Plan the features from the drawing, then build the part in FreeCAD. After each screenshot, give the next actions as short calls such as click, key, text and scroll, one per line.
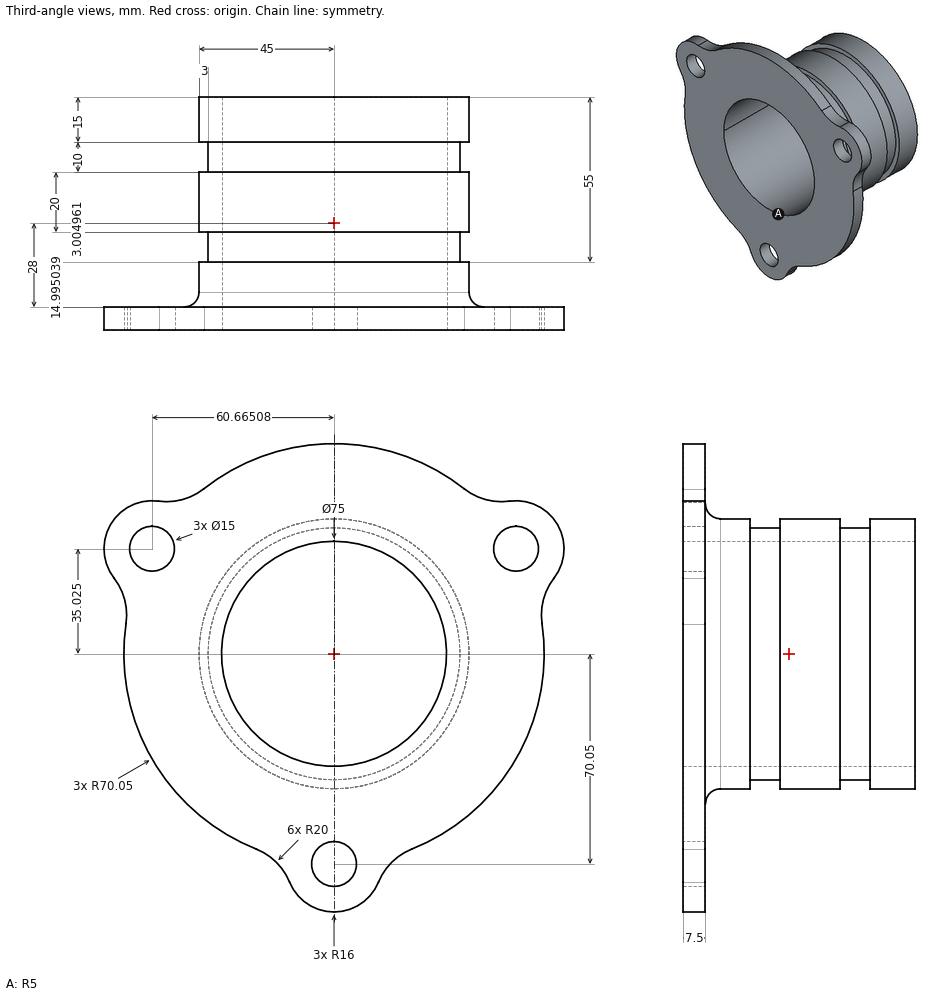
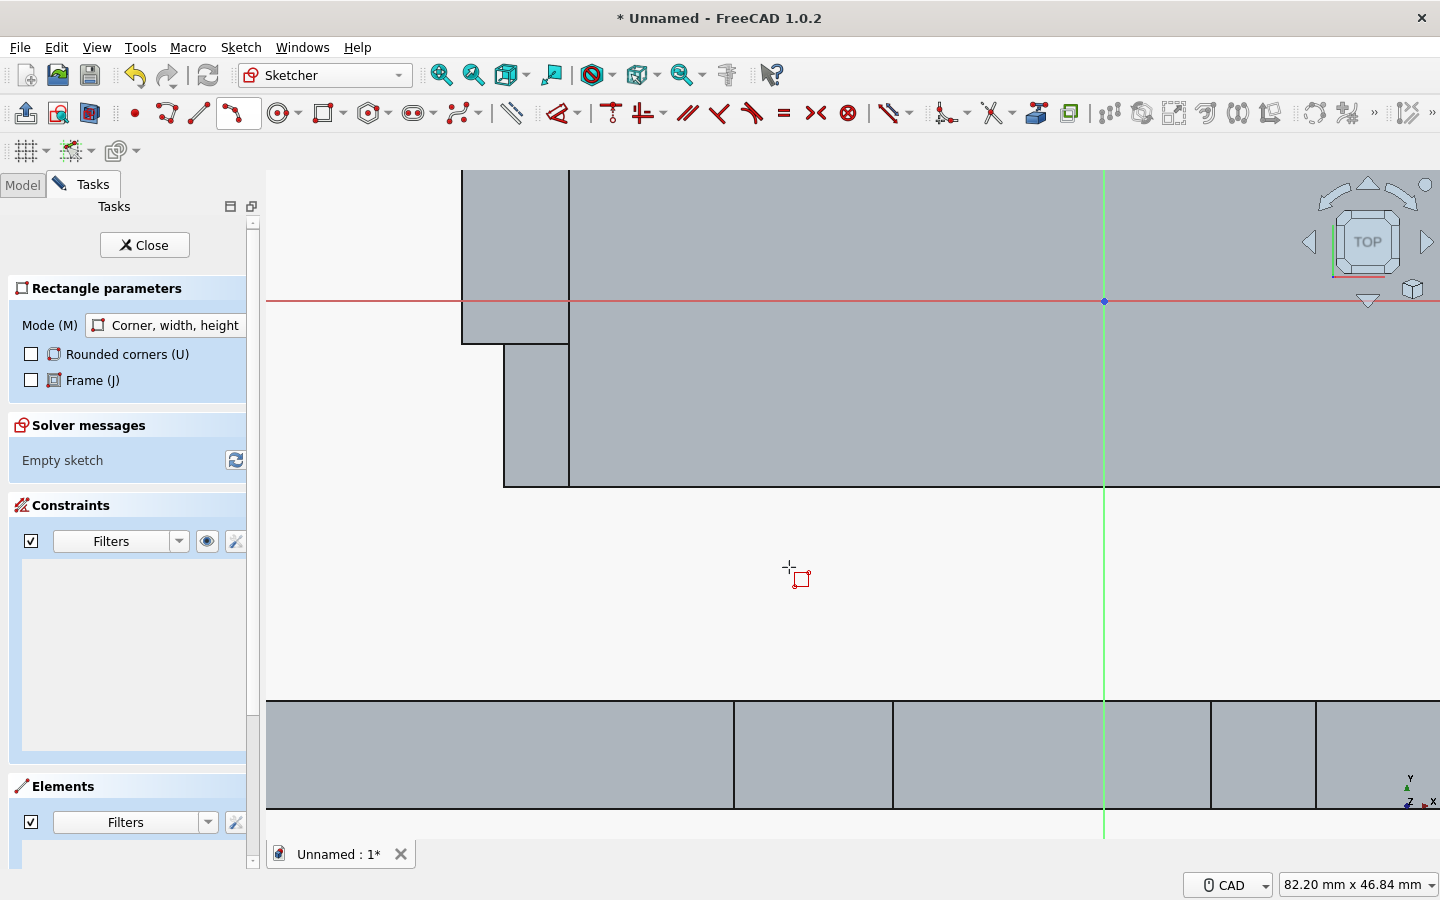
click(462, 487)
click(1104, 701)
key(Escape)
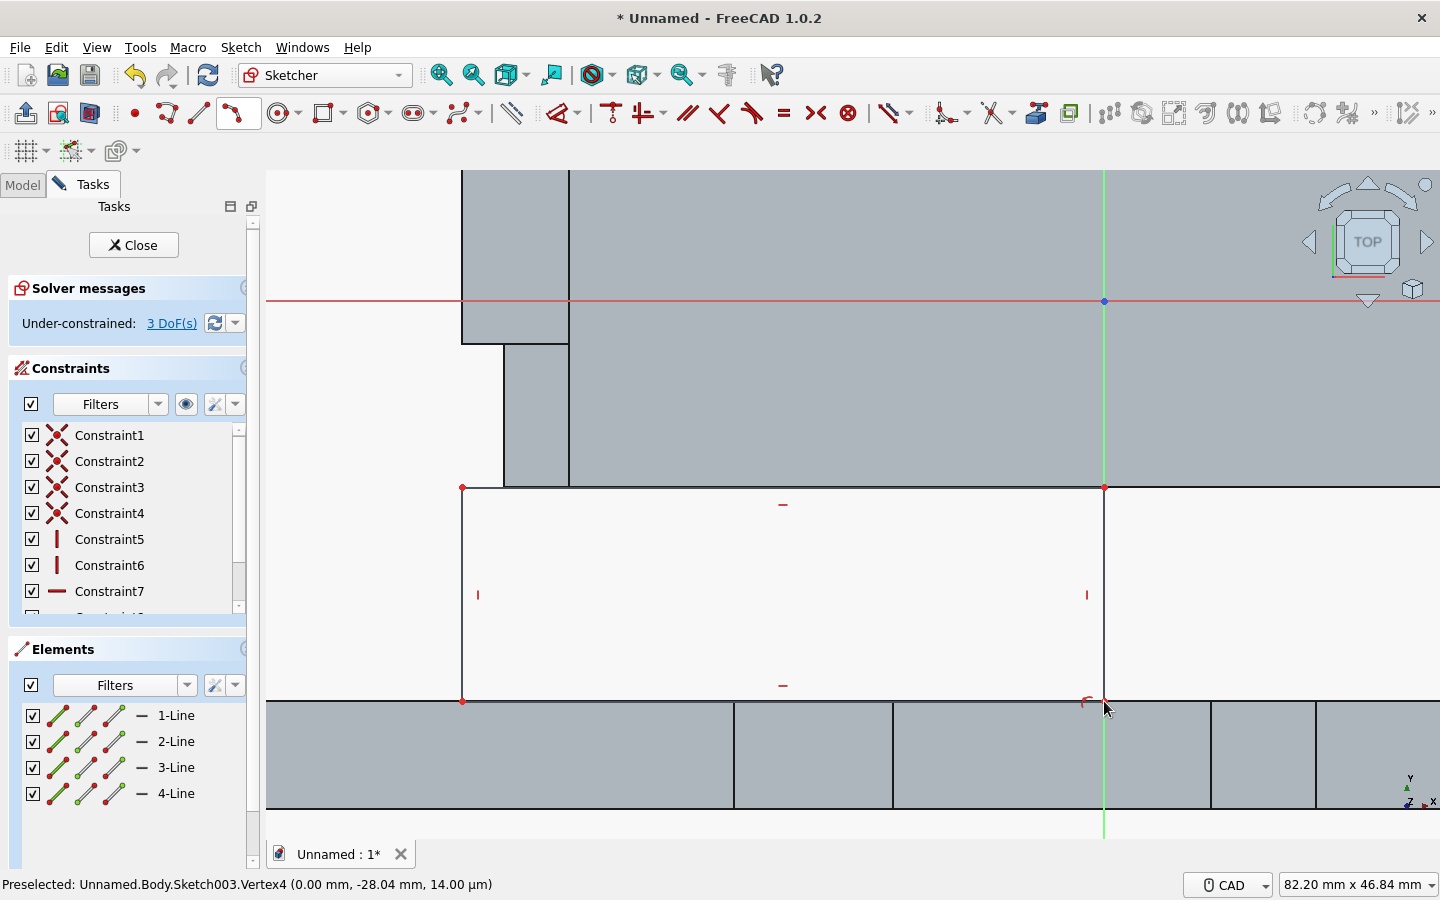
click(558, 114)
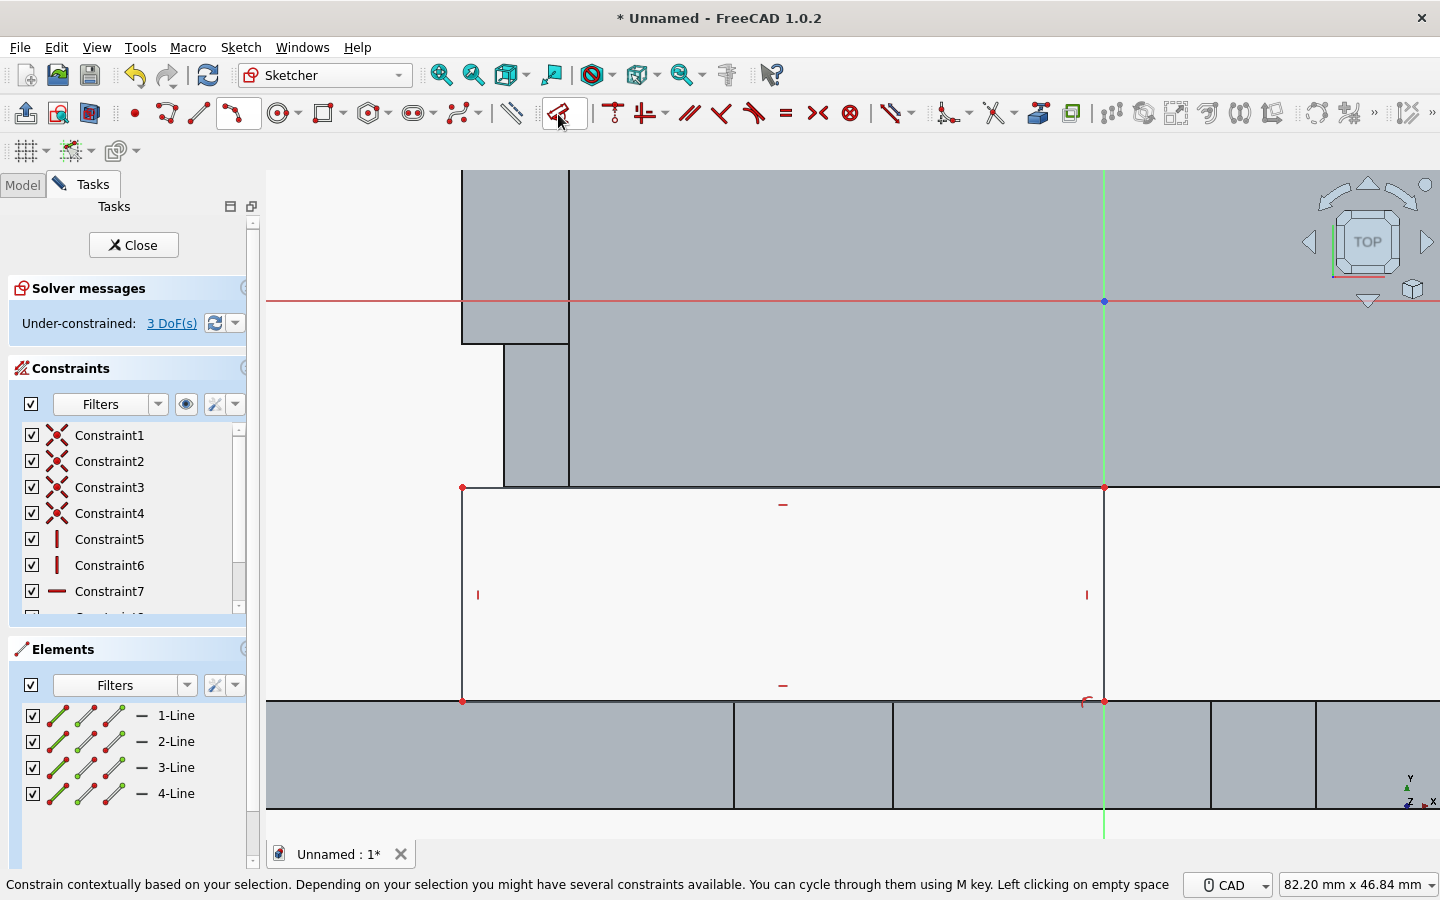
click(655, 702)
click(783, 736)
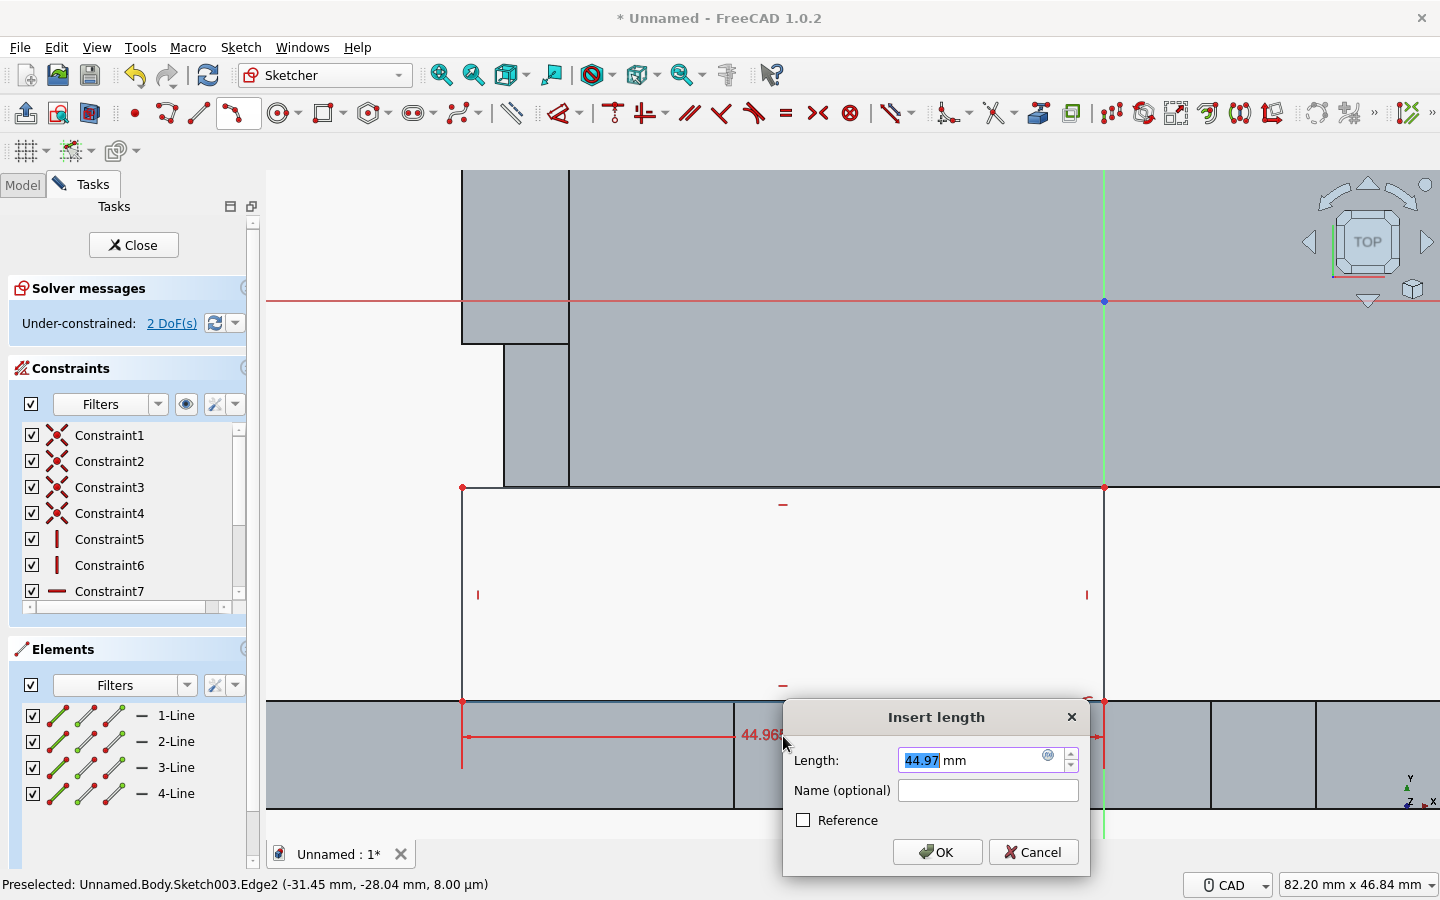
text(45)
key(Return)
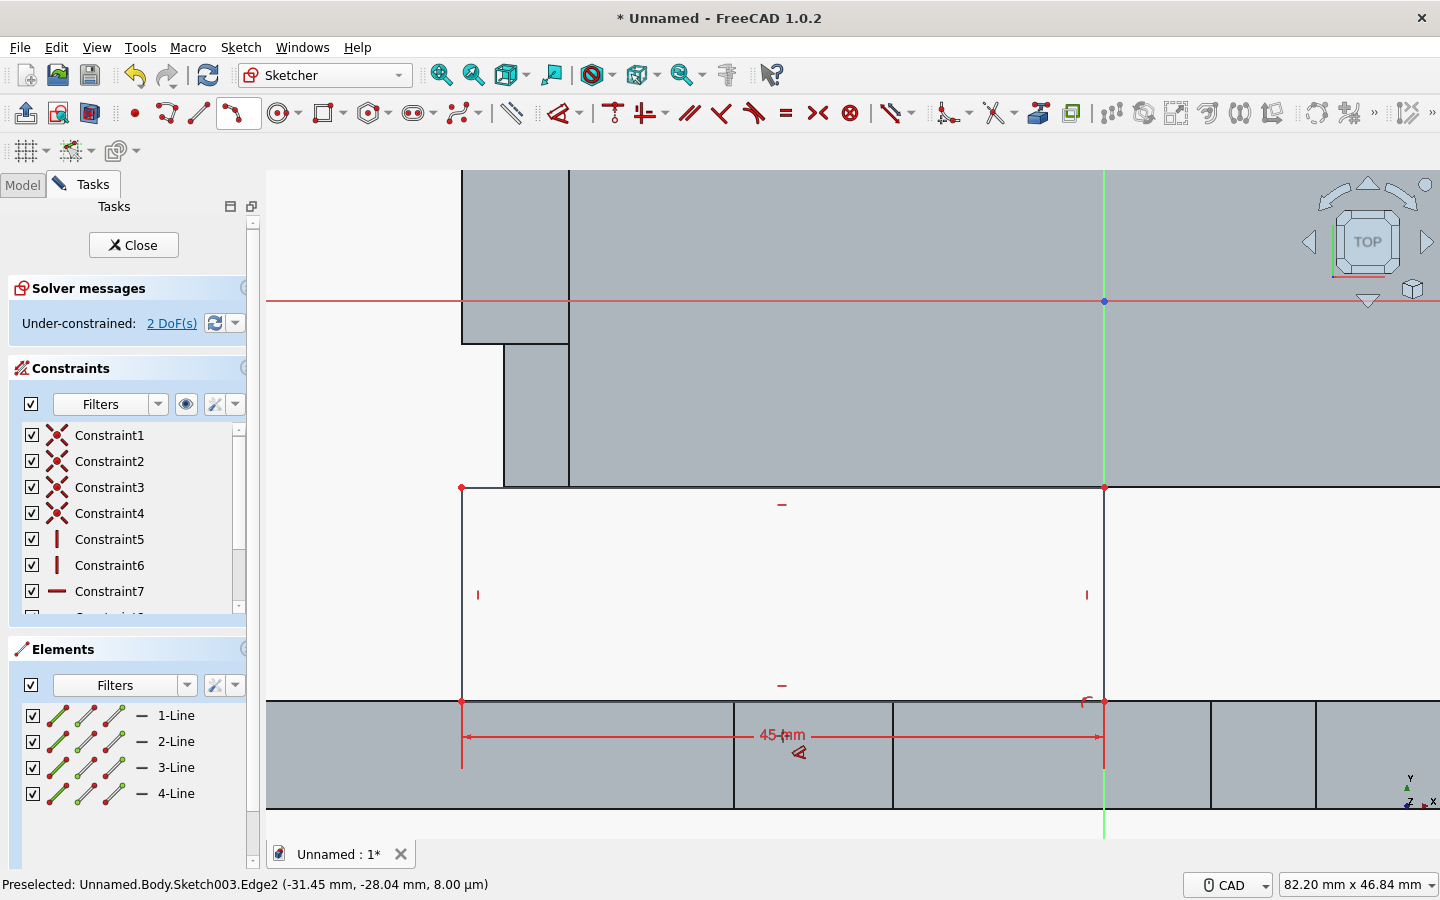
click(462, 702)
click(1138, 502)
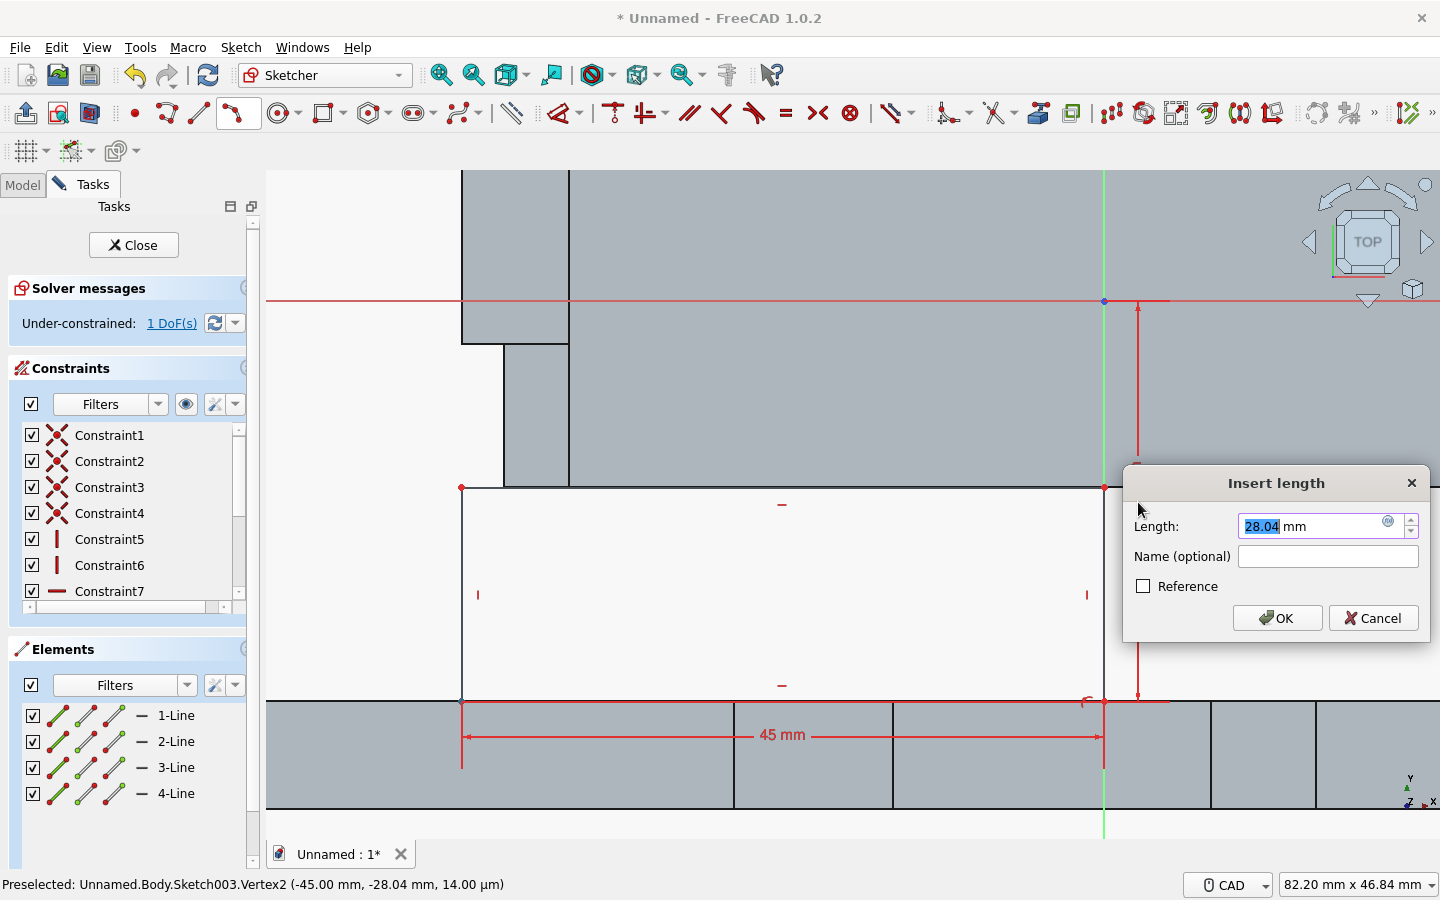
text(28)
key(Return)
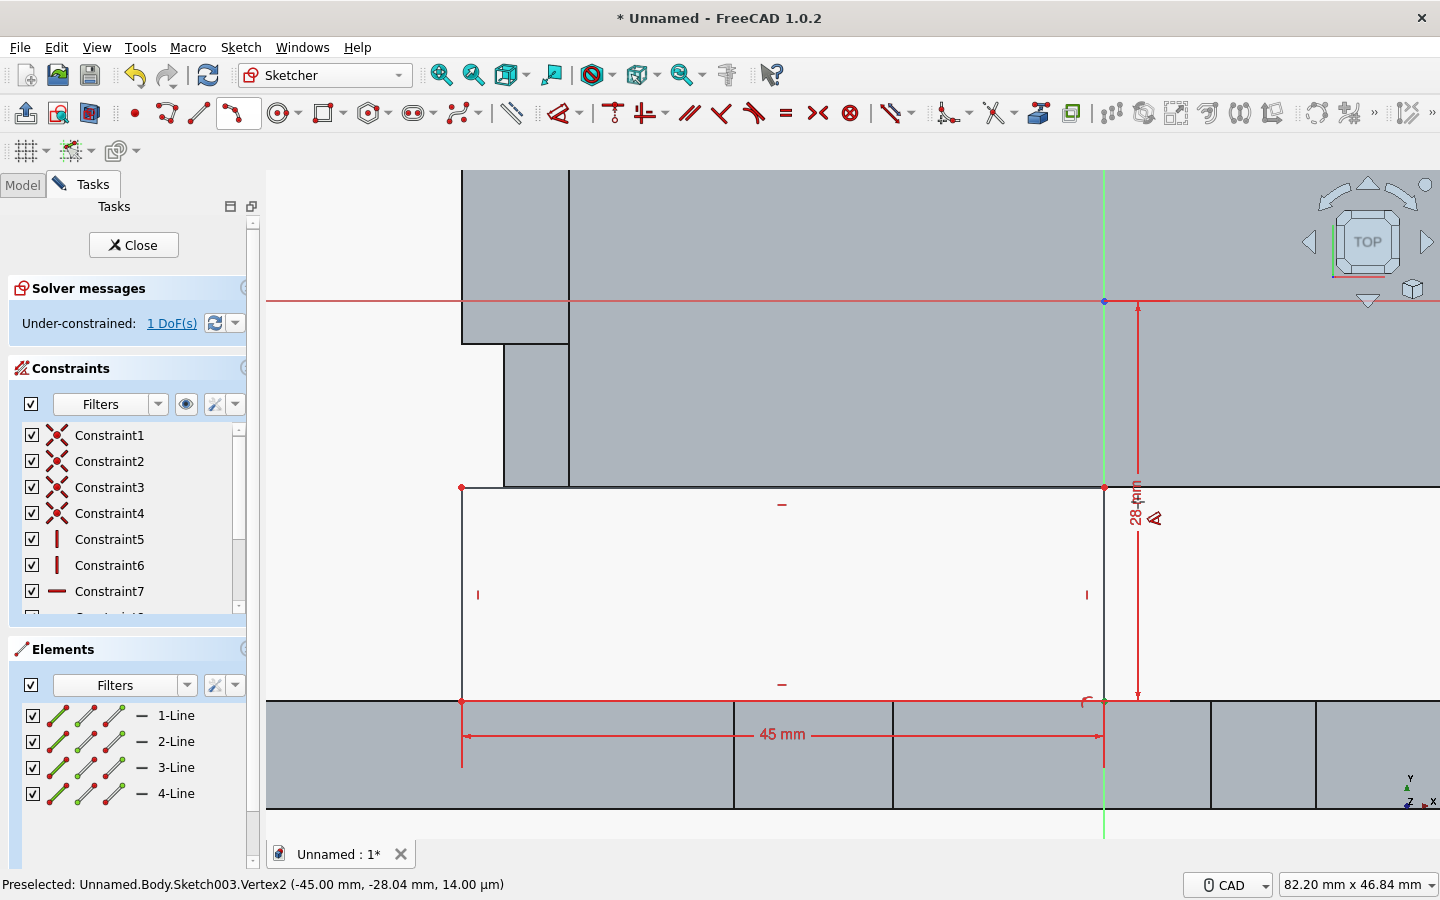
click(462, 552)
click(428, 595)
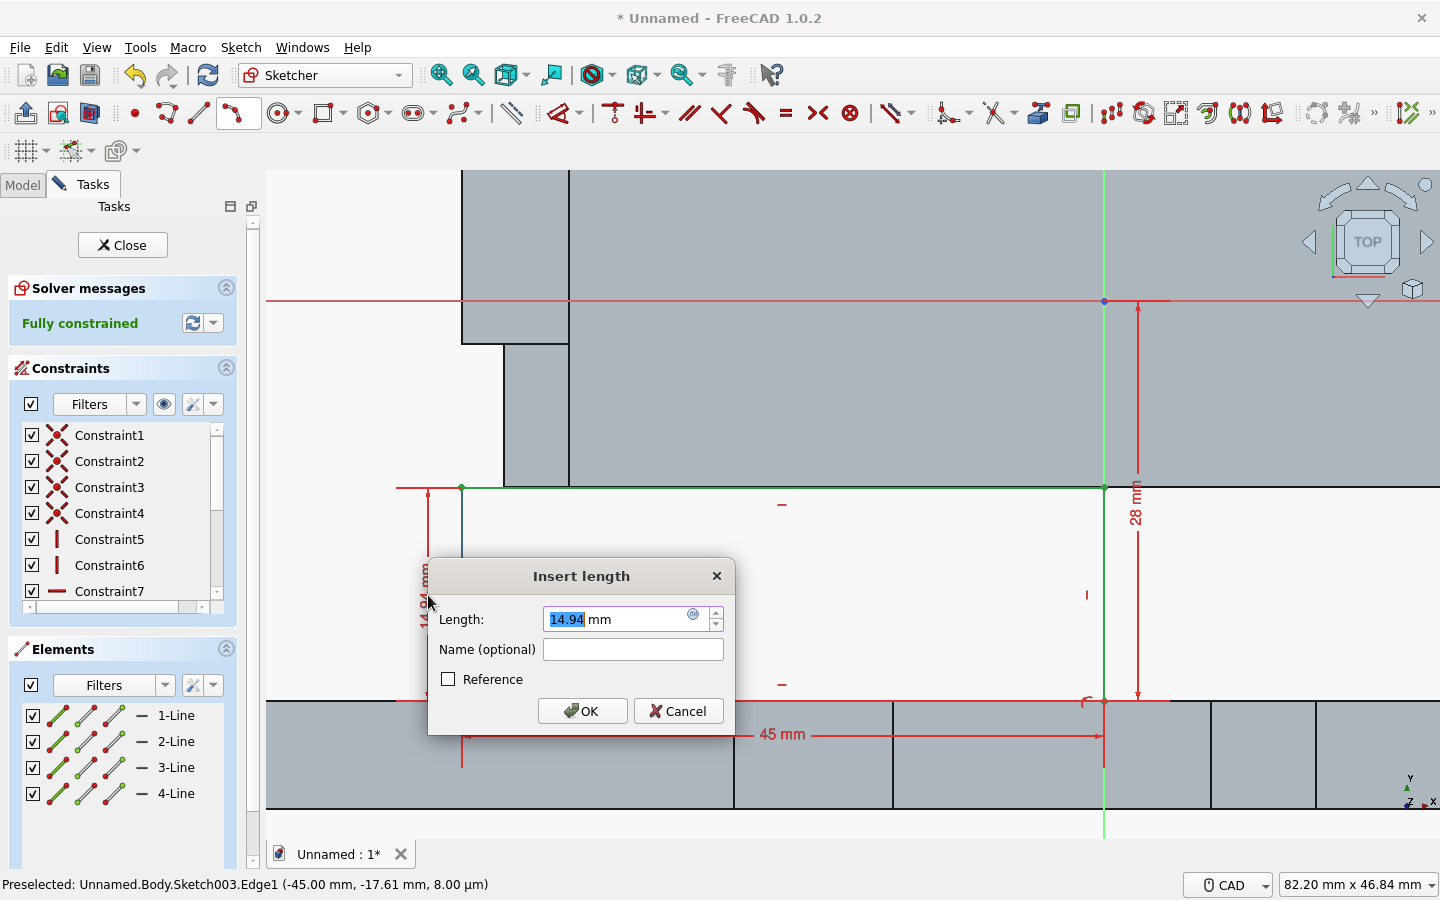
text(14.995039)
key(Return)
key(Escape)